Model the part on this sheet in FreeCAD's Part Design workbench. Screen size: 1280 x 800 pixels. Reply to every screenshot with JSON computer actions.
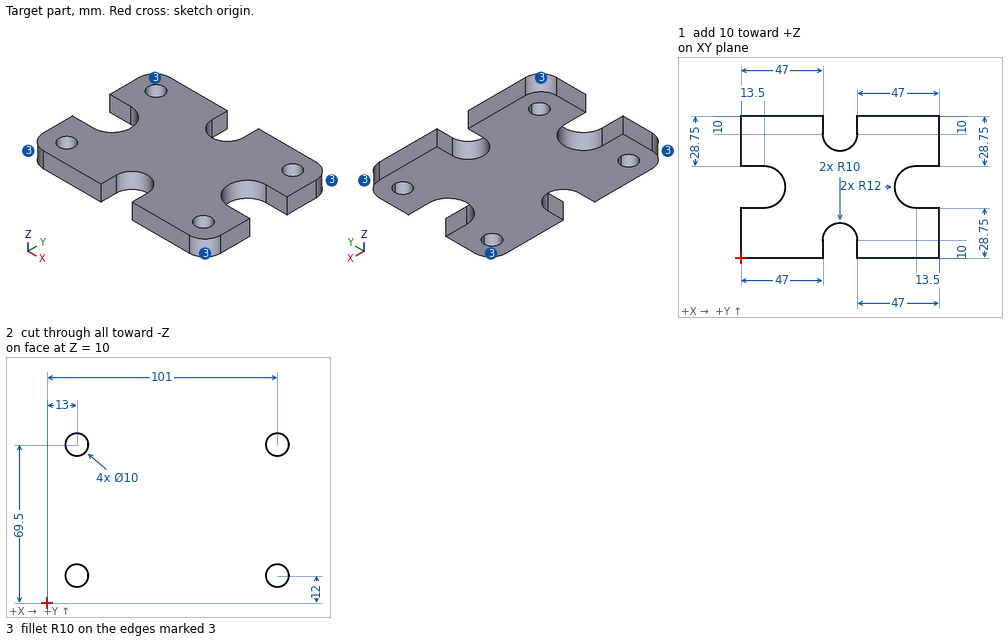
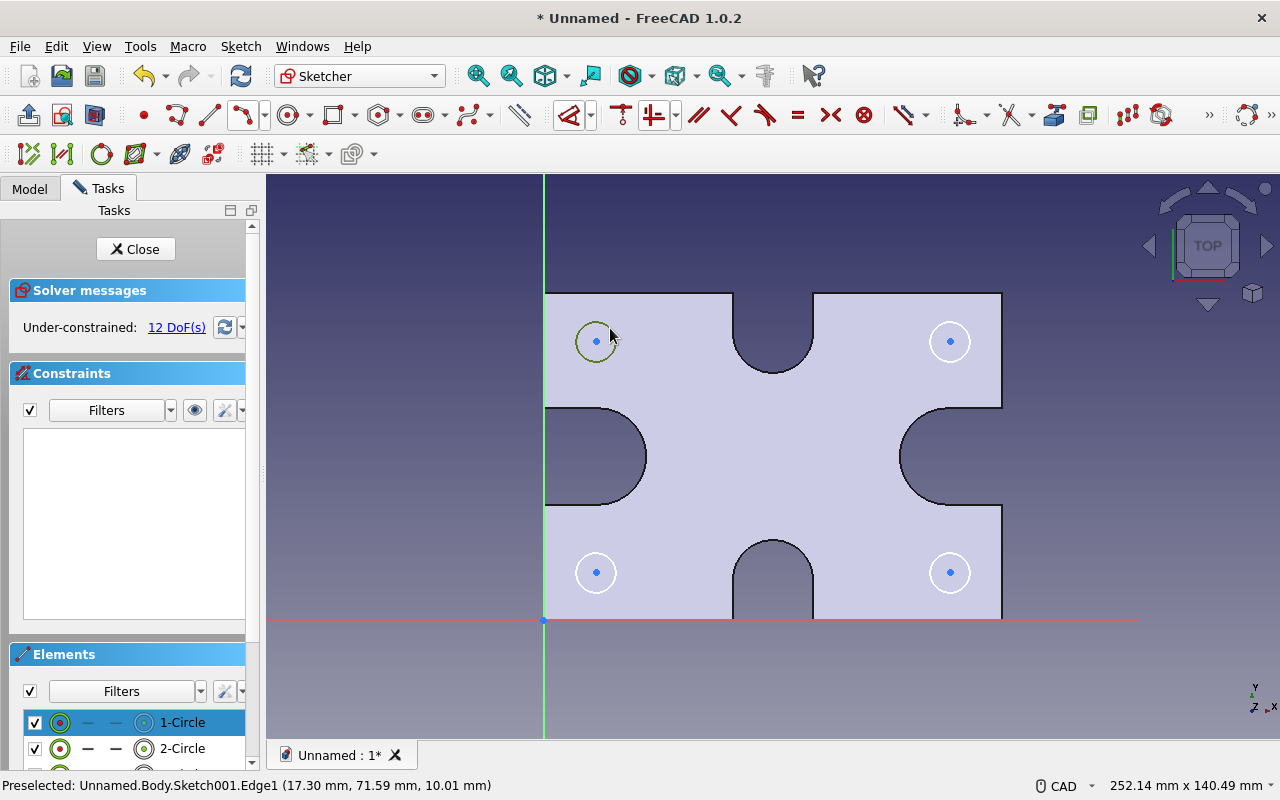
{"action": "left_click", "coordinate": [964, 328]}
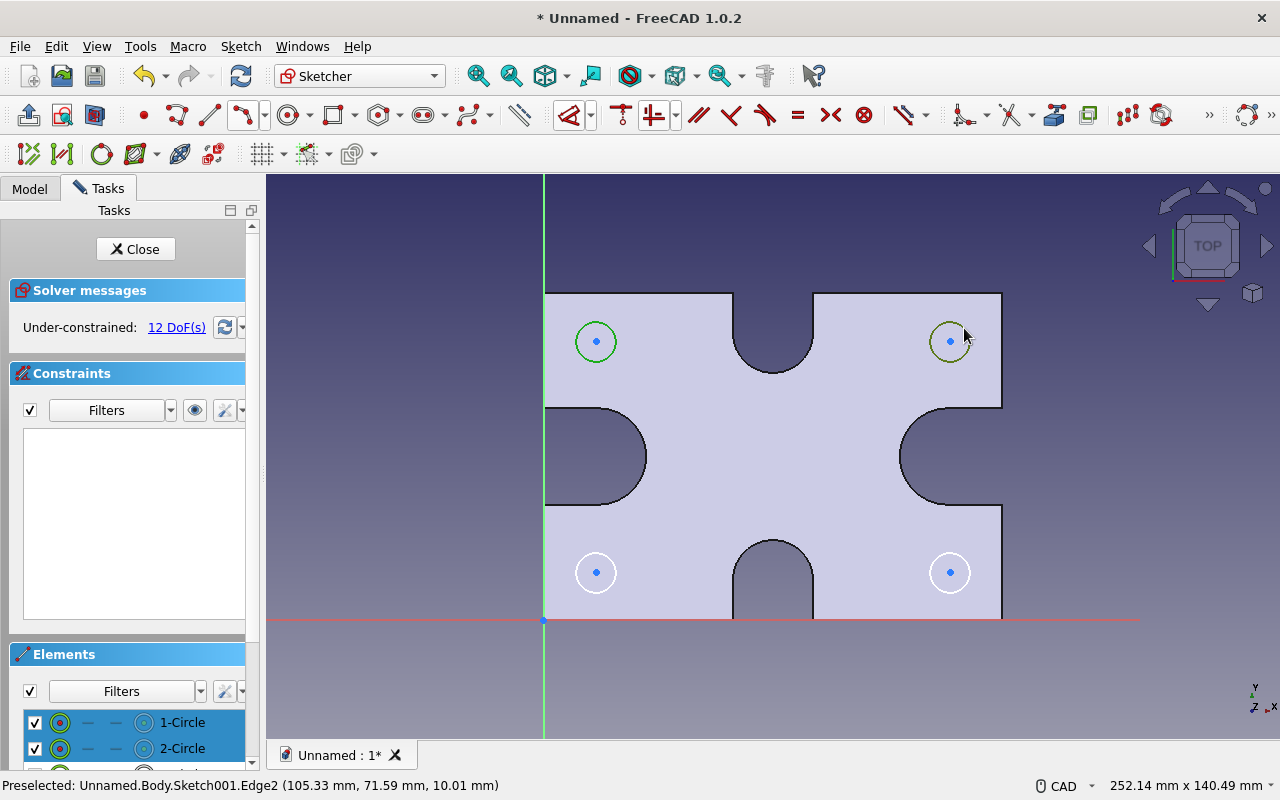
{"action": "left_click", "coordinate": [964, 559]}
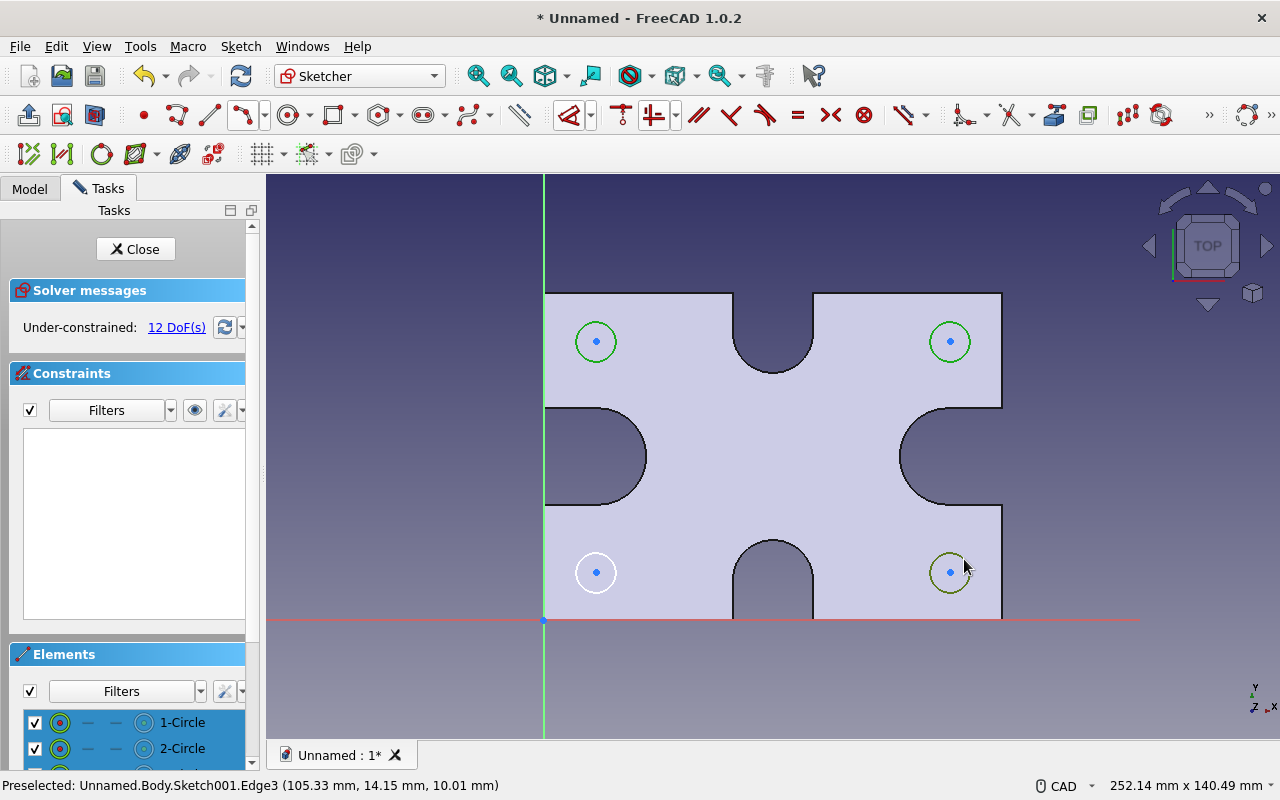
{"action": "left_click", "coordinate": [610, 559]}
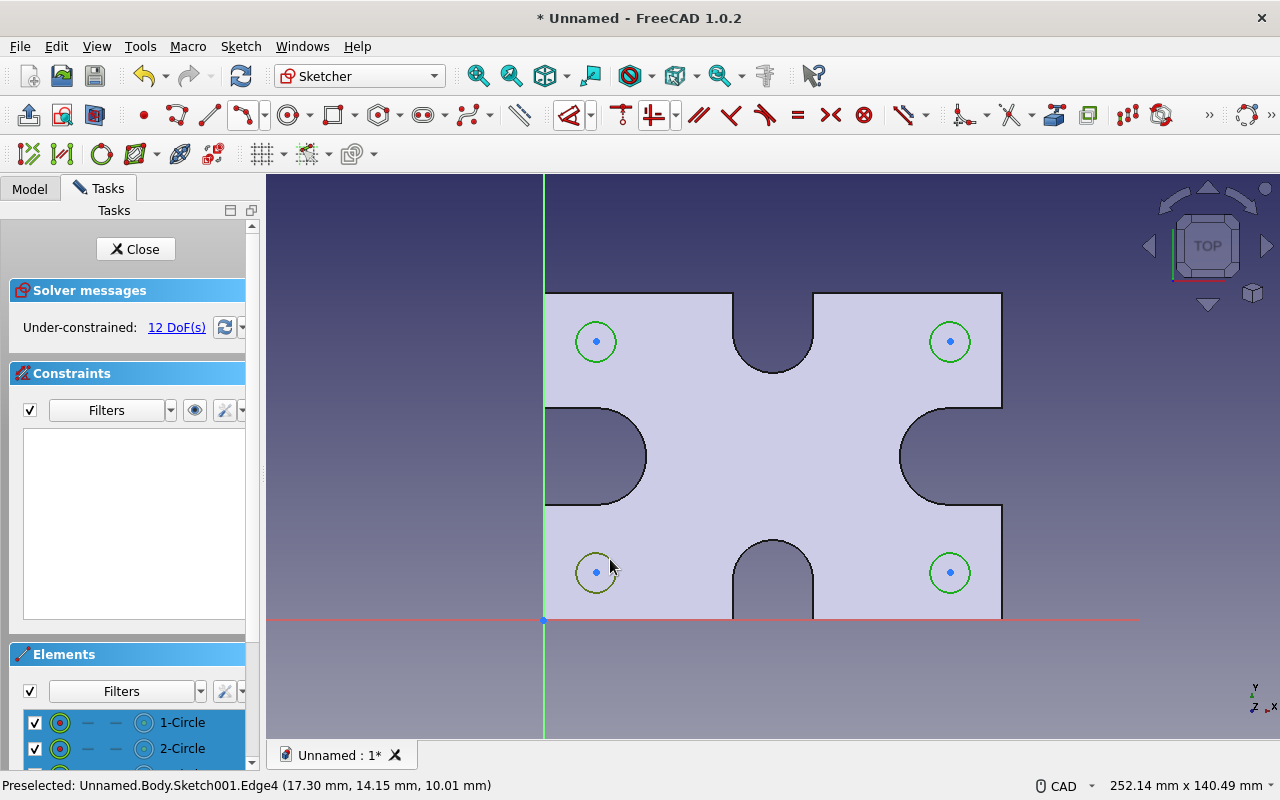
{"action": "left_click", "coordinate": [798, 116]}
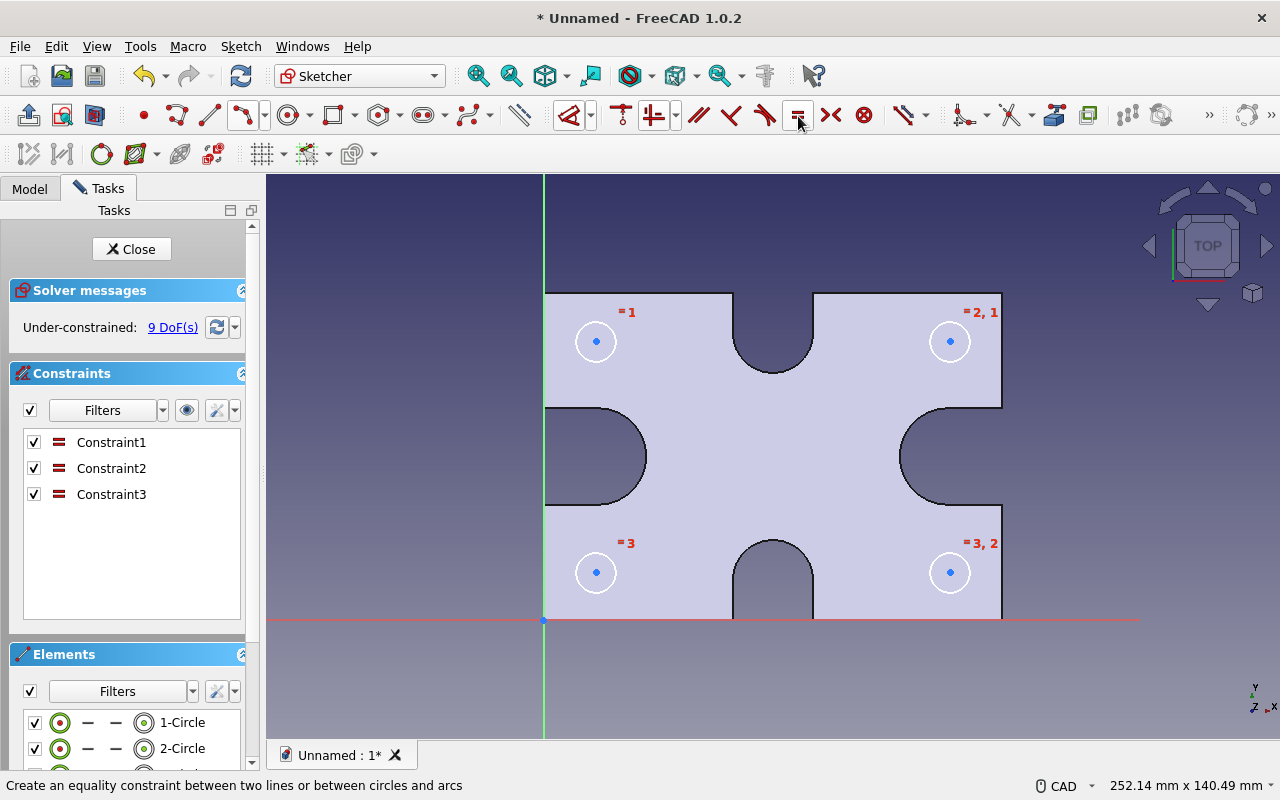
{"action": "left_click", "coordinate": [596, 342]}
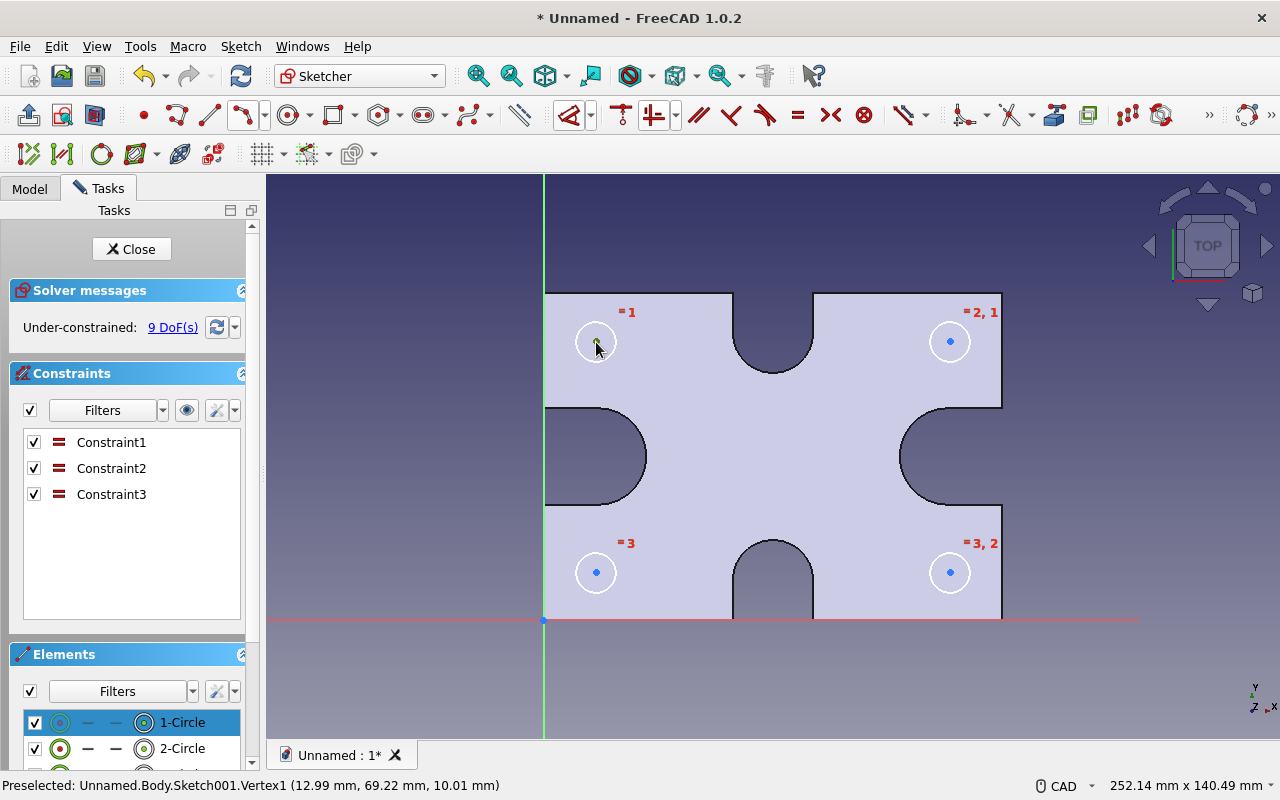
{"action": "left_click", "coordinate": [950, 342]}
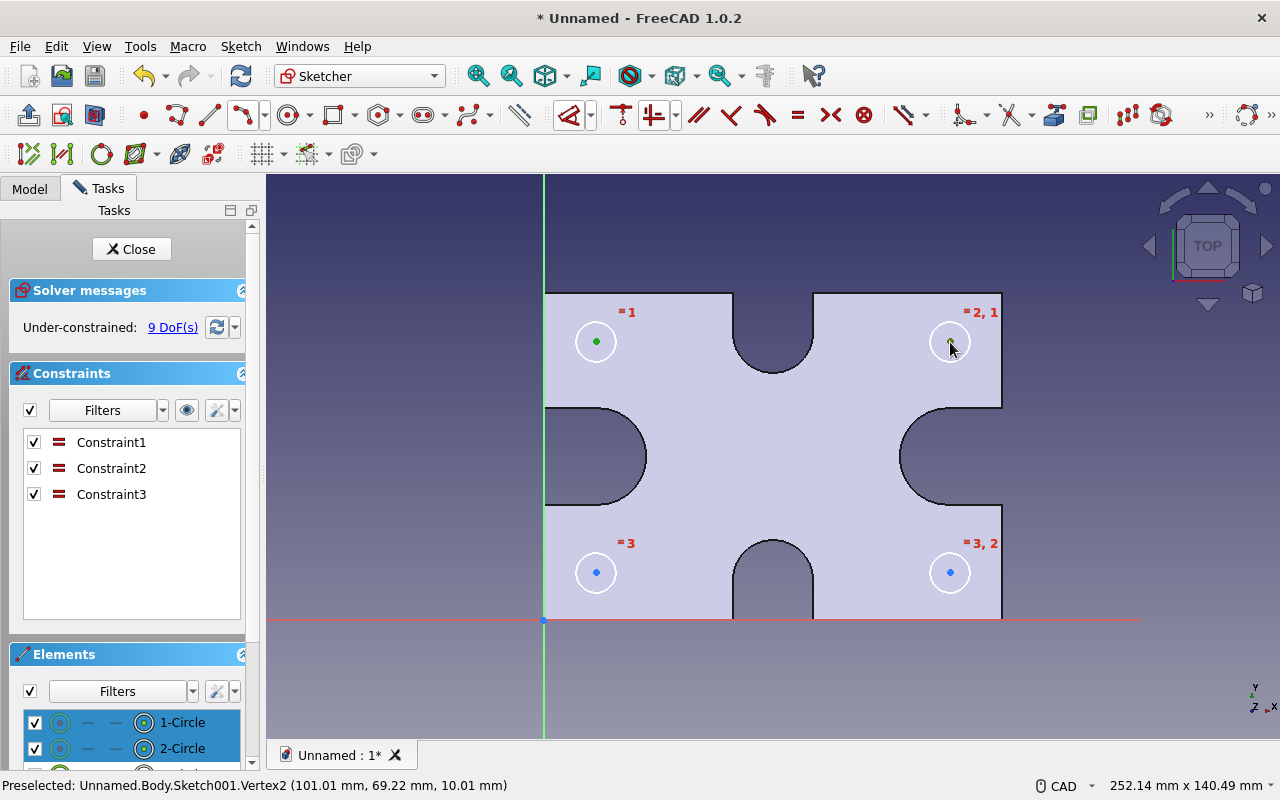
{"action": "left_click", "coordinate": [676, 116]}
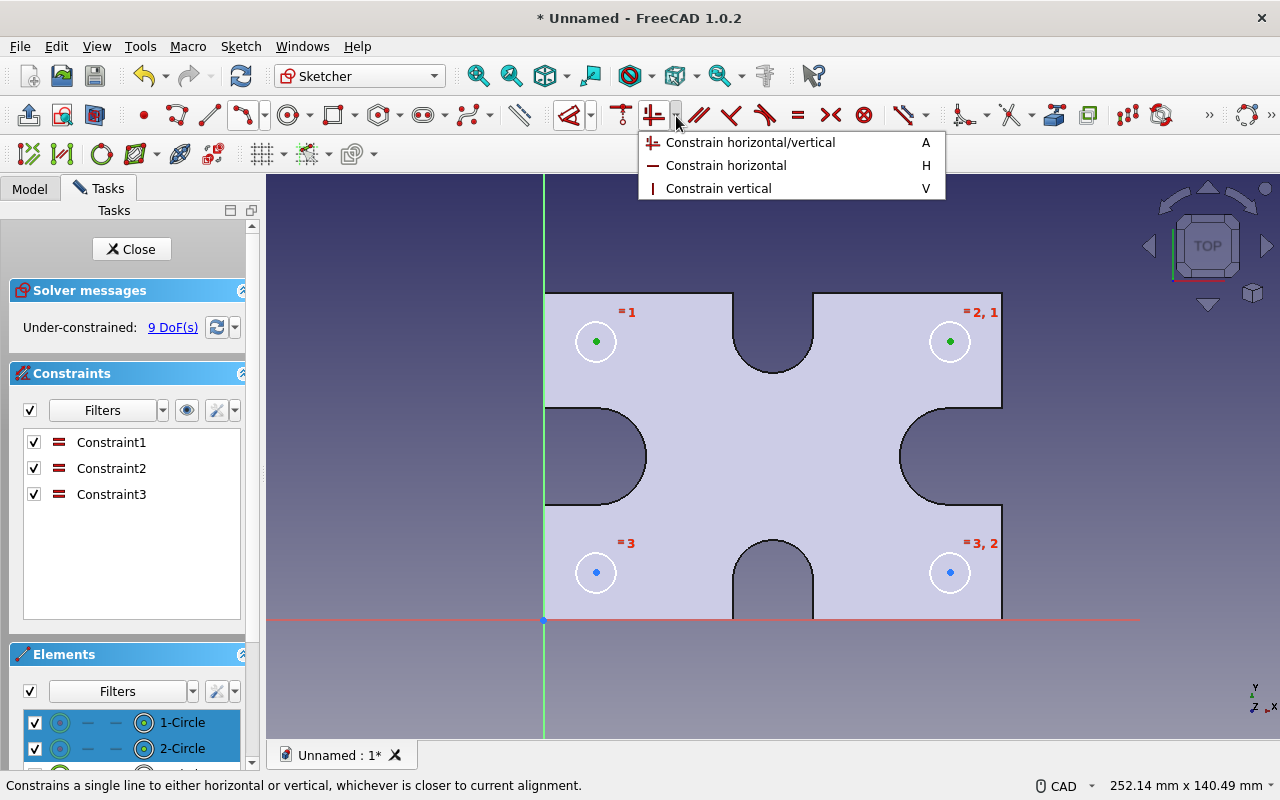
{"action": "left_click", "coordinate": [792, 166]}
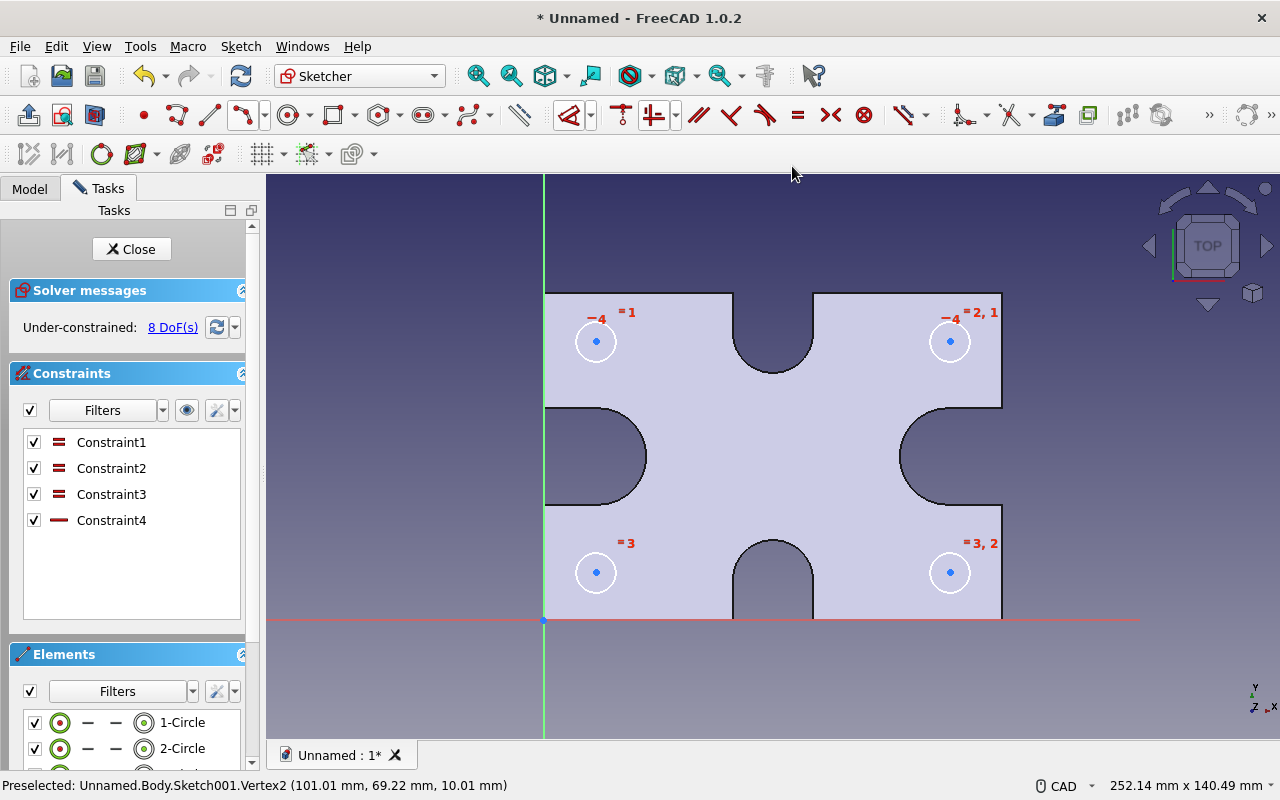
{"action": "left_click", "coordinate": [950, 342]}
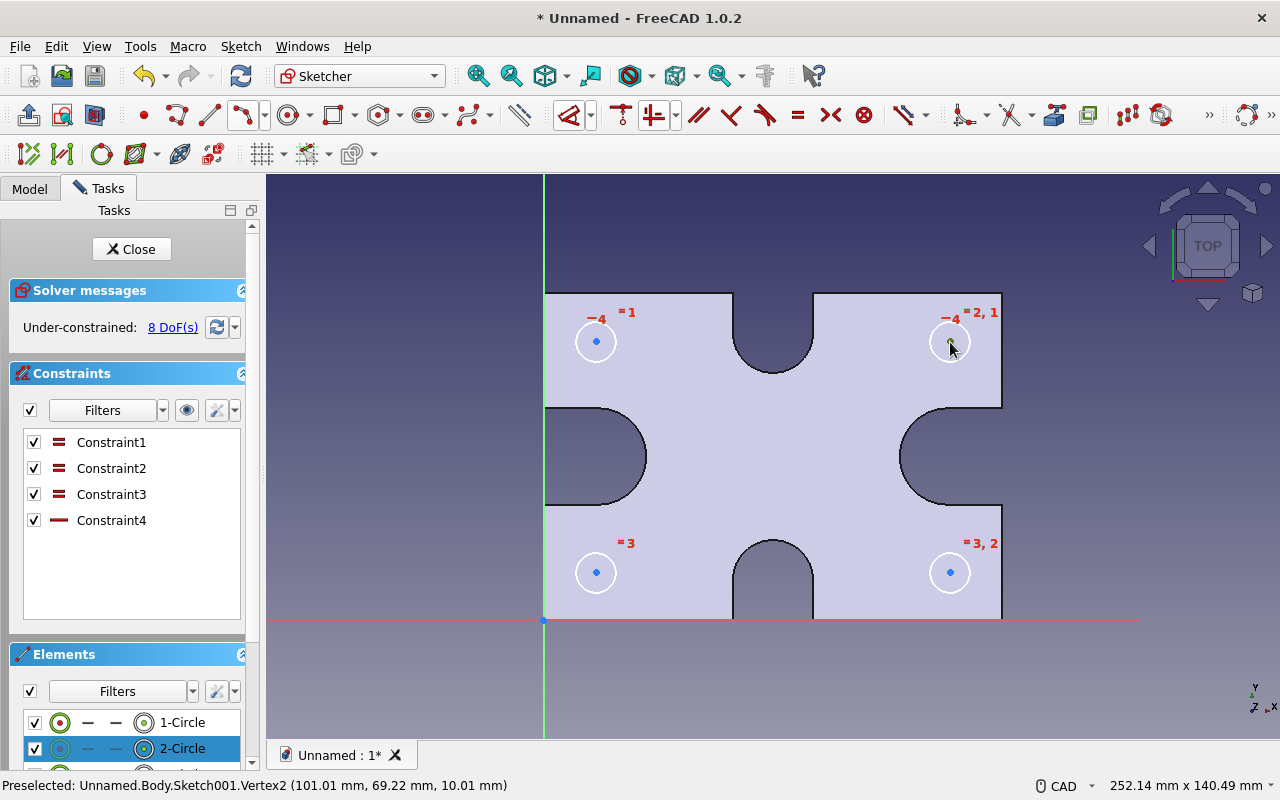
{"action": "left_click", "coordinate": [950, 573]}